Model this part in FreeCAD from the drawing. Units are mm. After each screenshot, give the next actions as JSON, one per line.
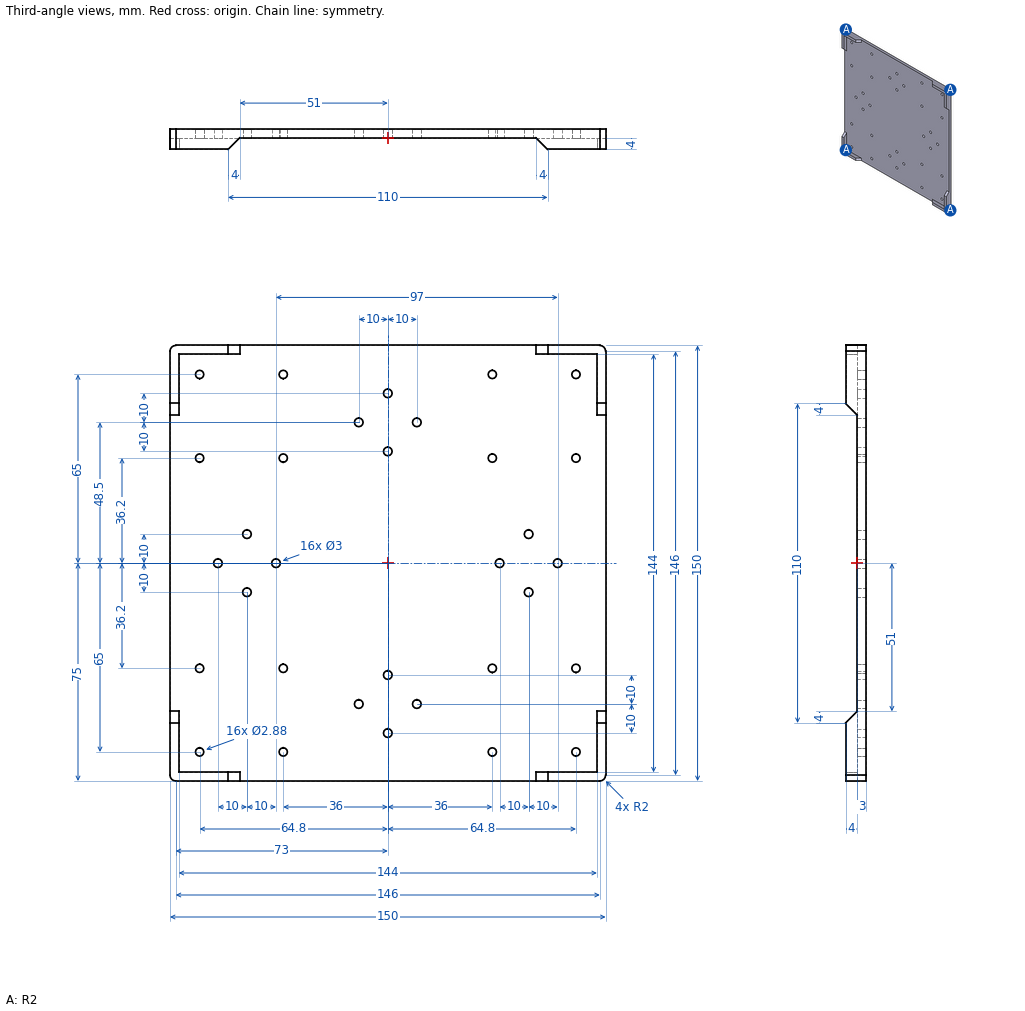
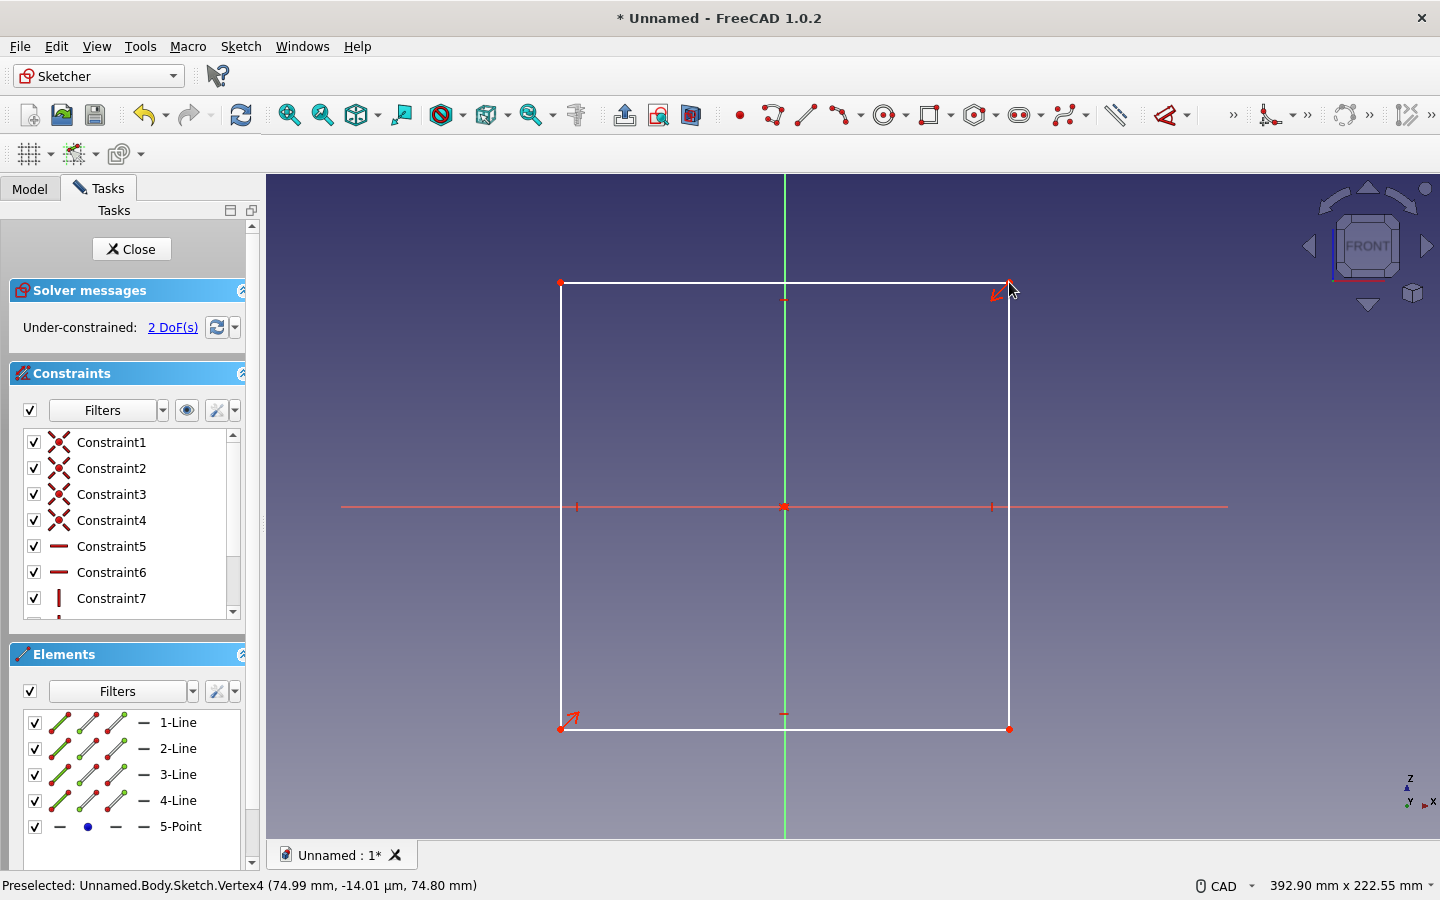
{"action": "key", "text": "d"}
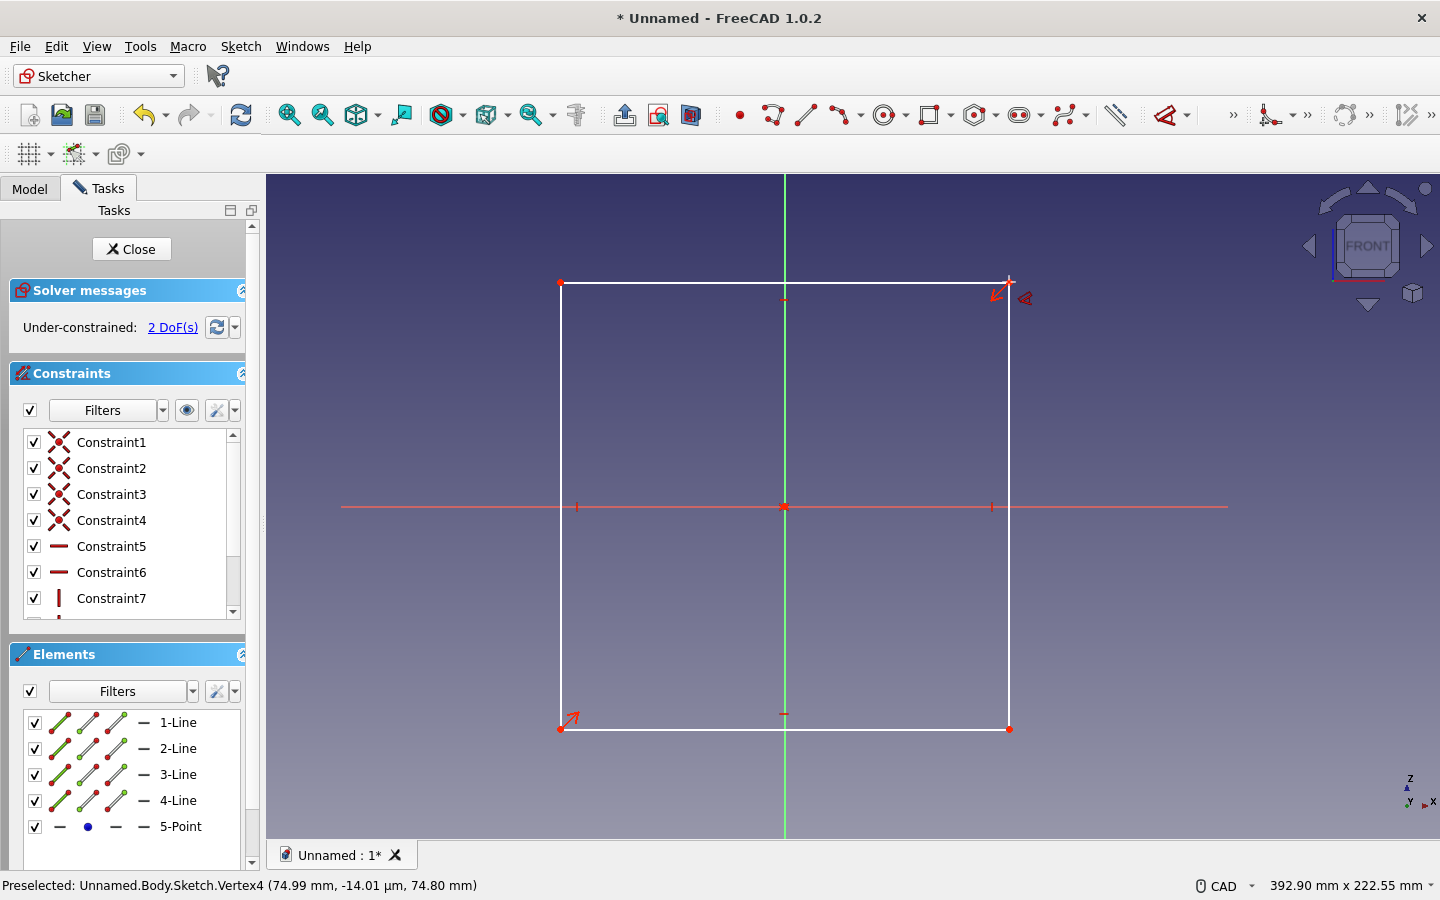
{"action": "left_click", "coordinate": [695, 730]}
{"action": "left_click", "coordinate": [682, 764]}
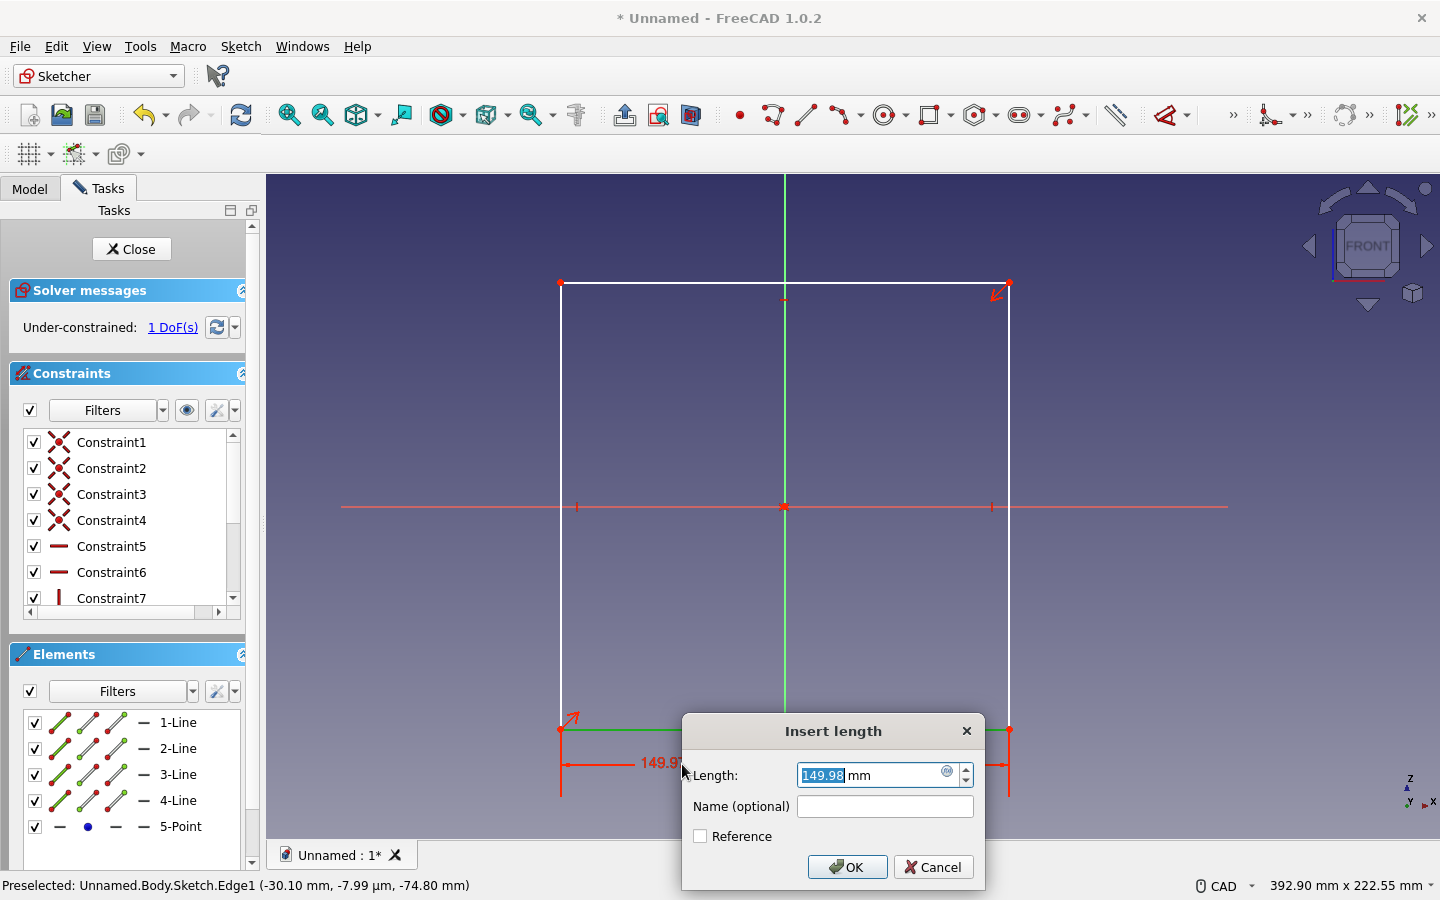
{"action": "type", "text": "150"}
{"action": "key", "text": "Return"}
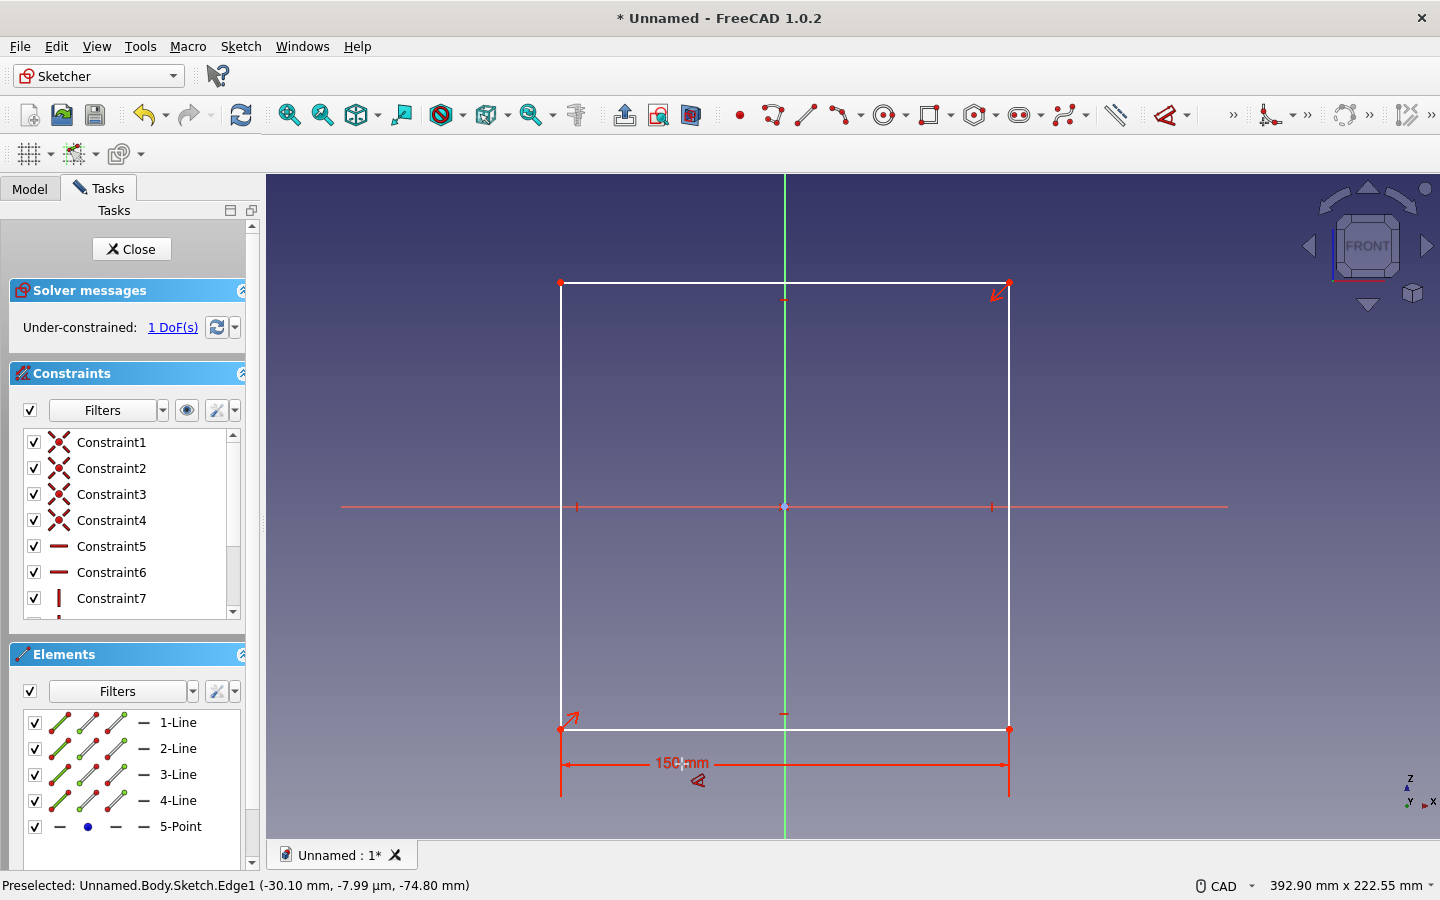
{"action": "left_click", "coordinate": [1009, 596]}
{"action": "left_click", "coordinate": [1043, 404]}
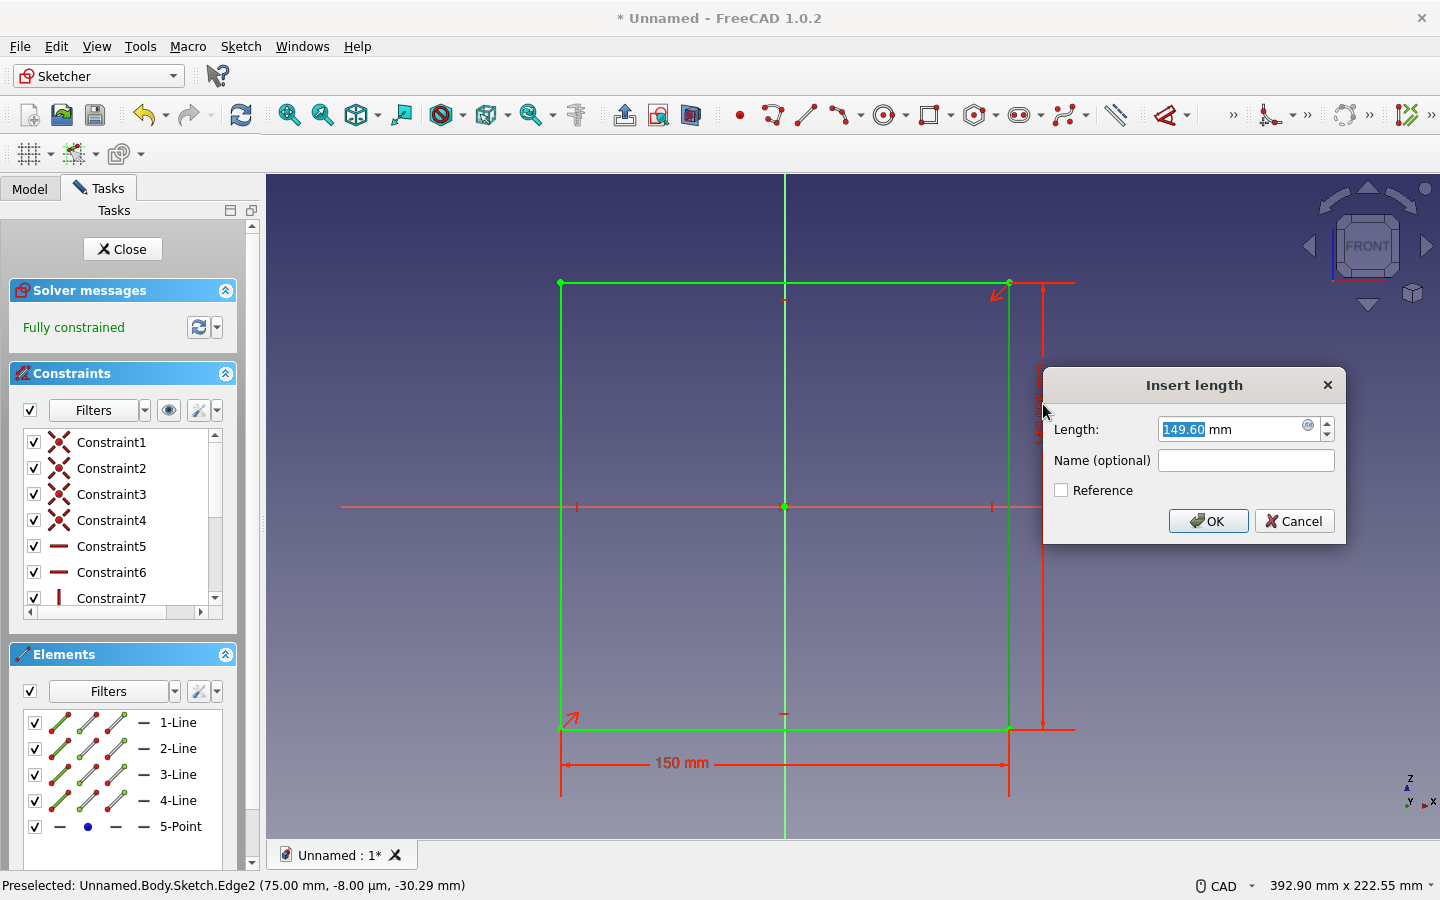
{"action": "type", "text": "150"}
{"action": "key", "text": "Return"}
{"action": "key", "text": "Escape"}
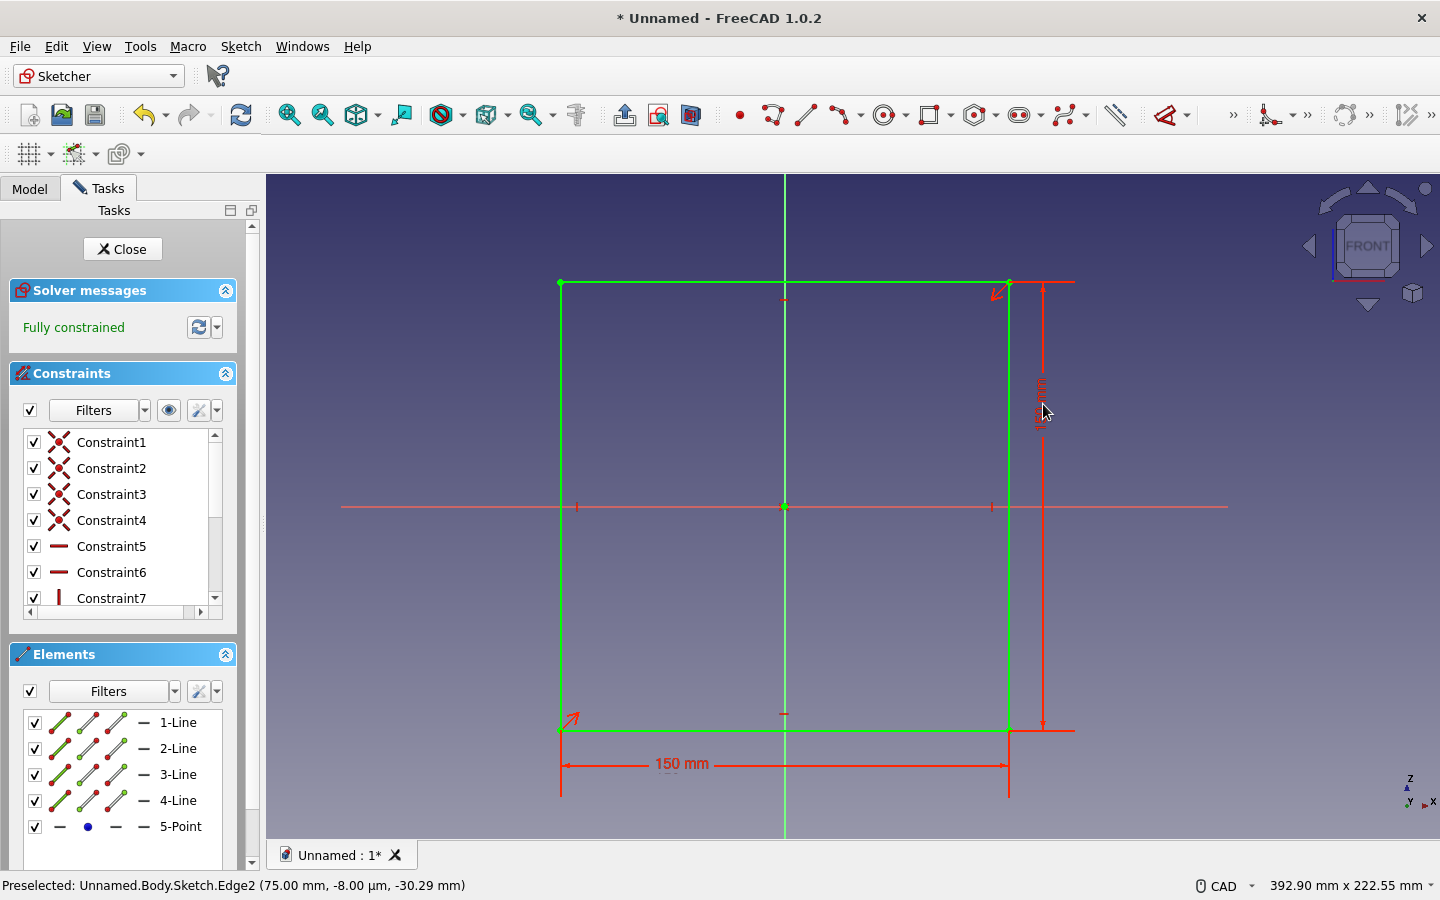
{"action": "left_click", "coordinate": [123, 249]}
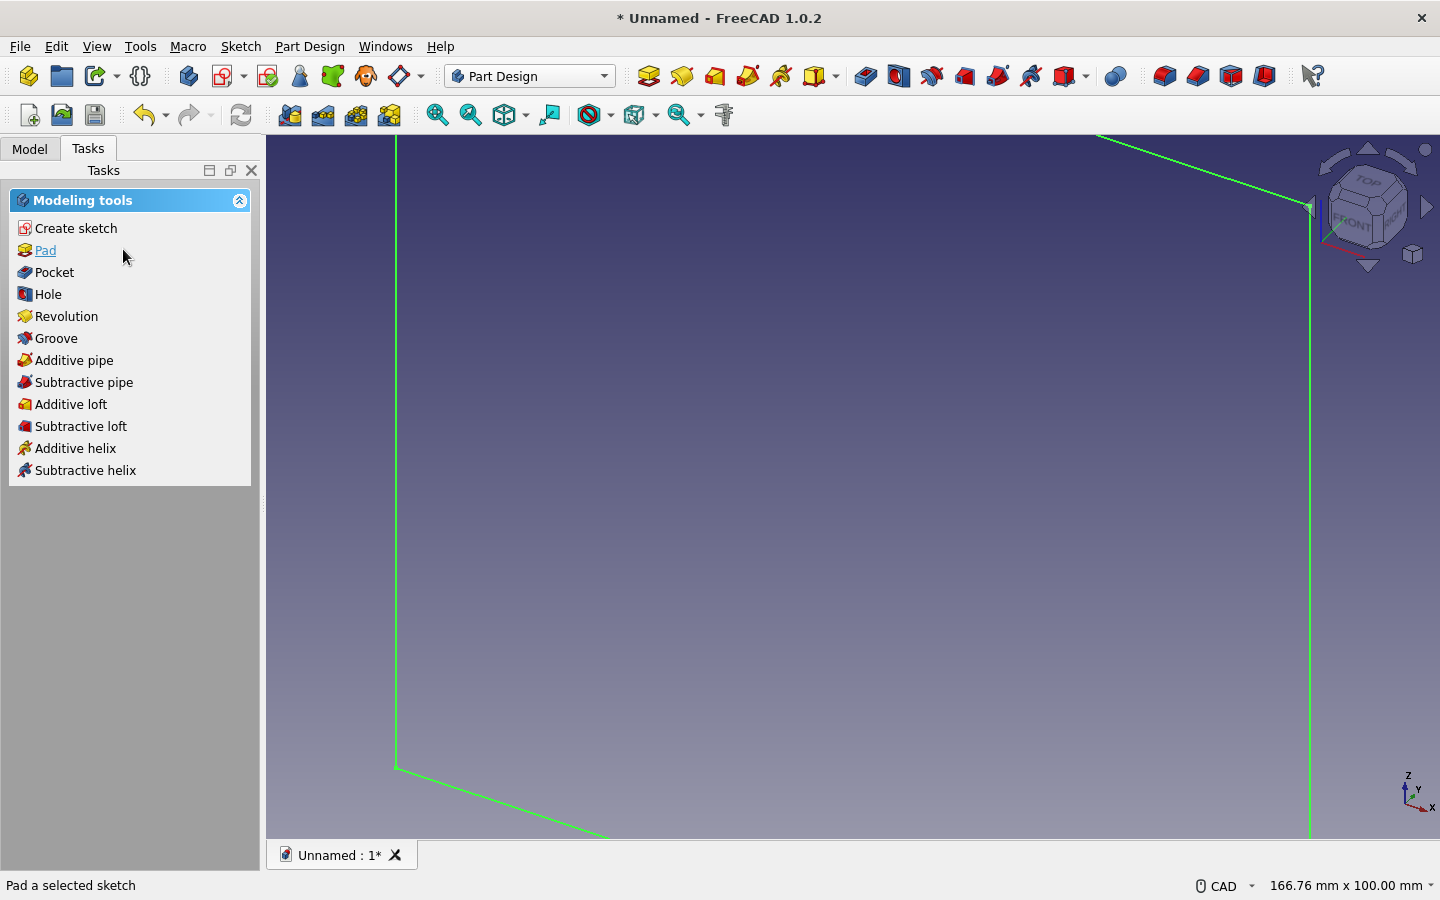
{"action": "left_click", "coordinate": [649, 76]}